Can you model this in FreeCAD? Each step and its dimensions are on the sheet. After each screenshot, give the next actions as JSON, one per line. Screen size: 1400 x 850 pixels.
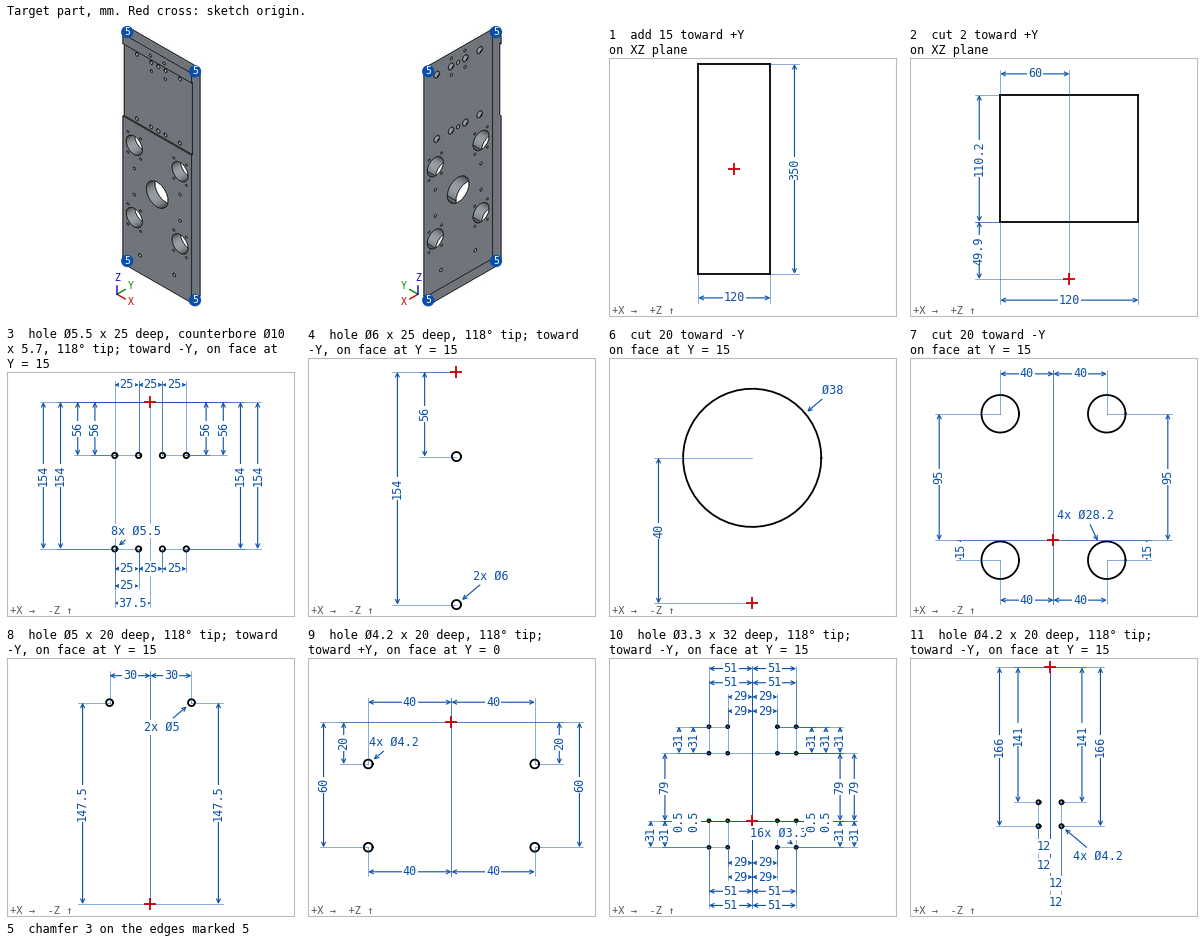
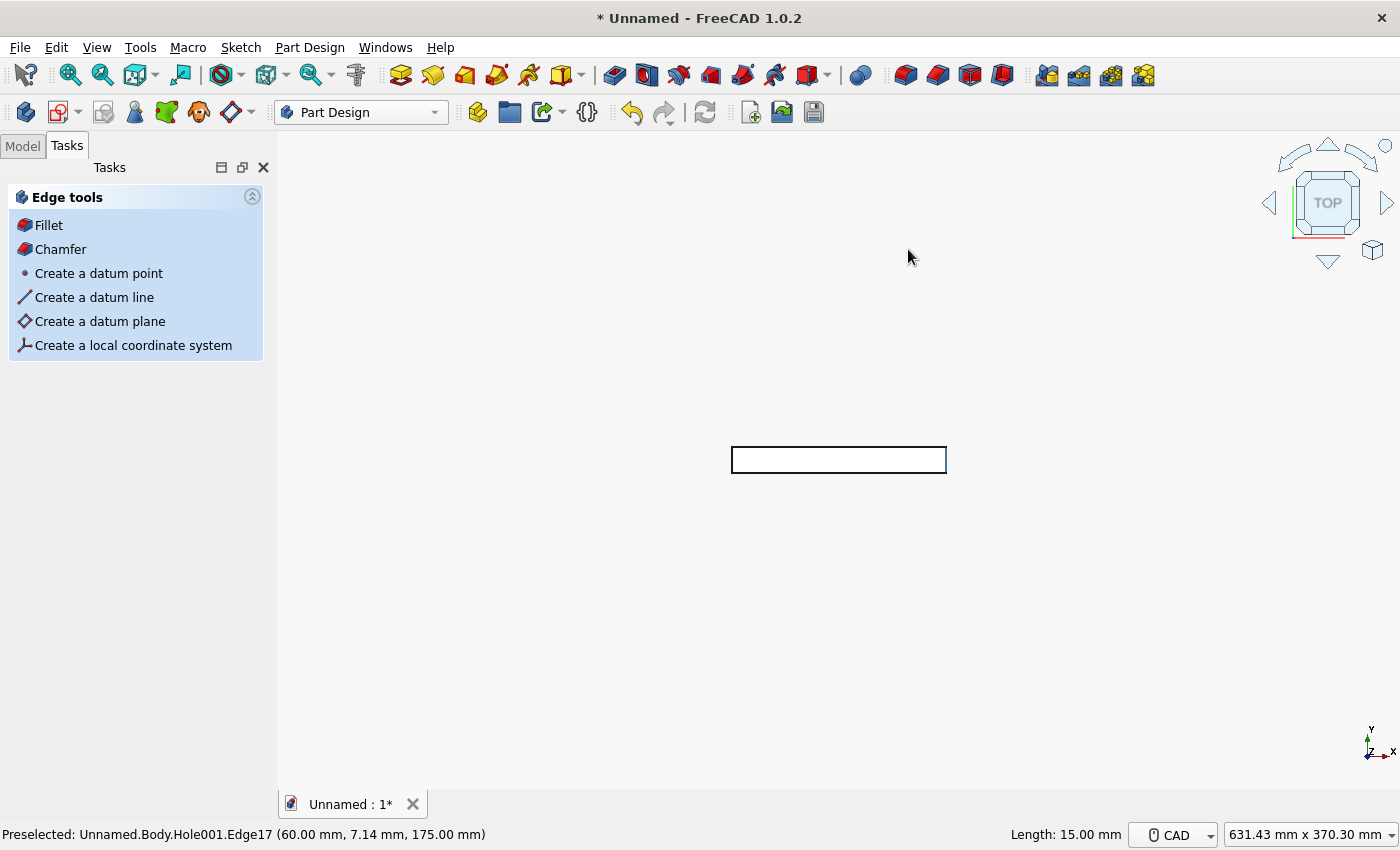
{"action": "key", "text": "v f"}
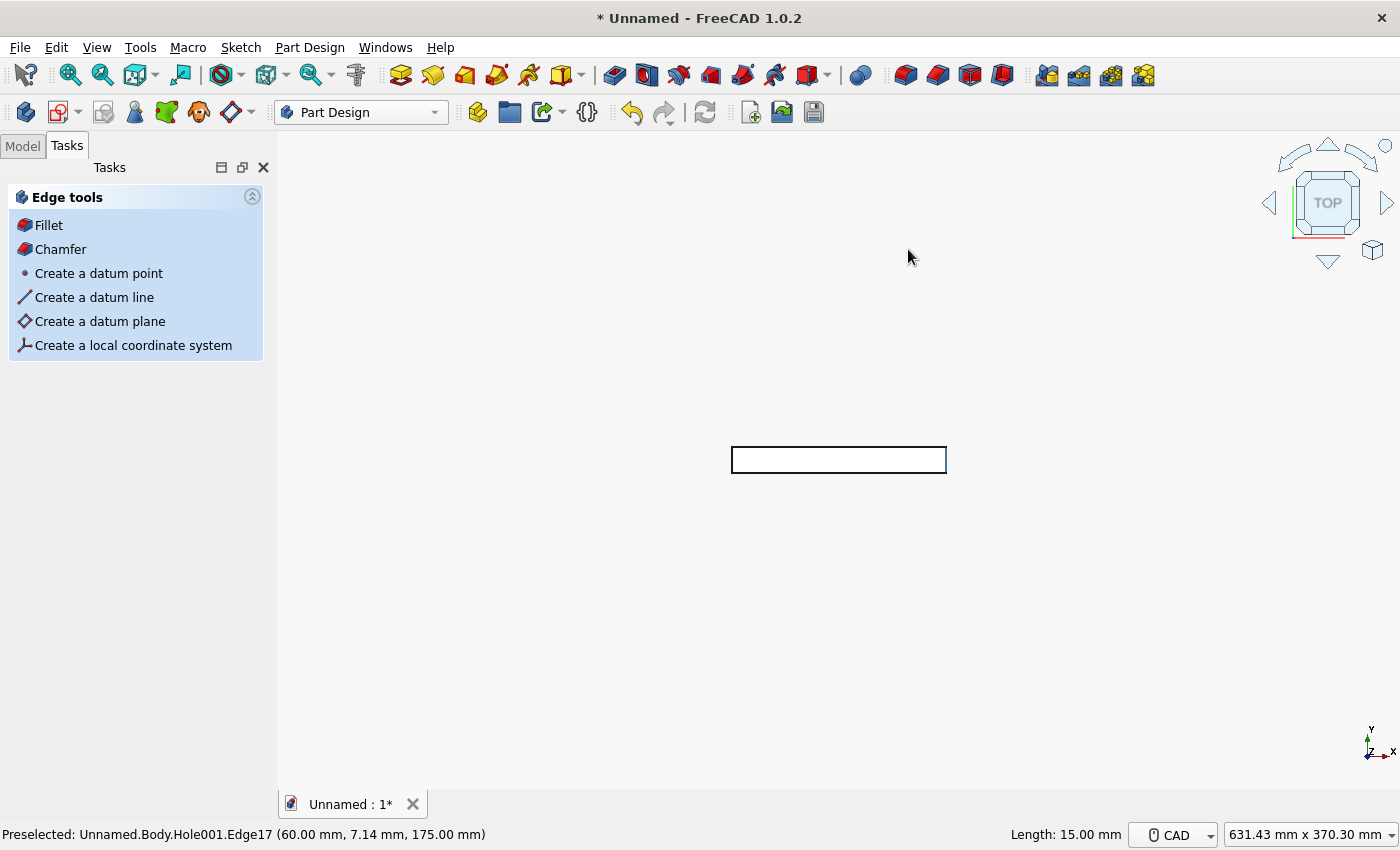
{"action": "left_click", "coordinate": [732, 459], "text": "ctrl"}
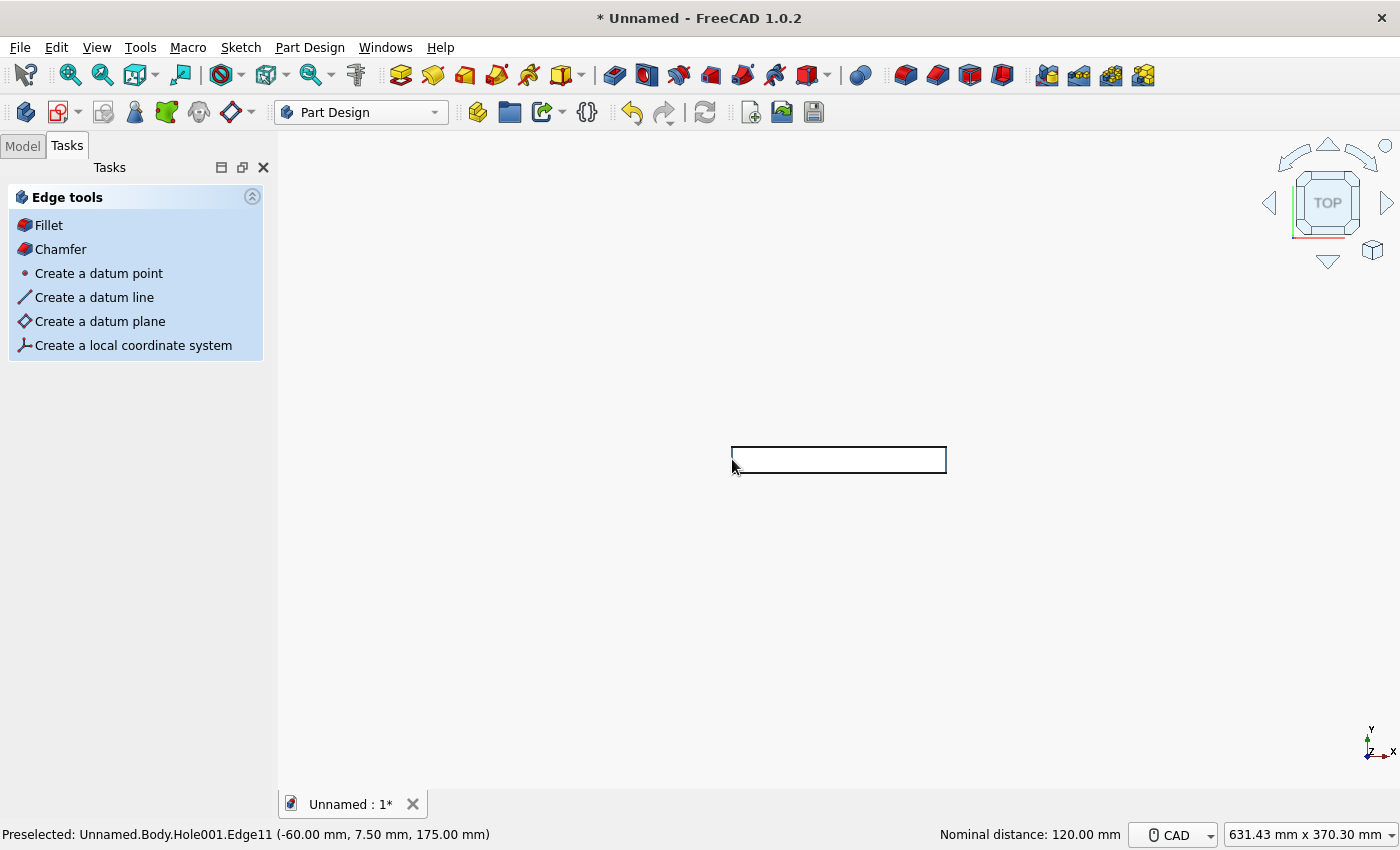
{"action": "key", "text": "1"}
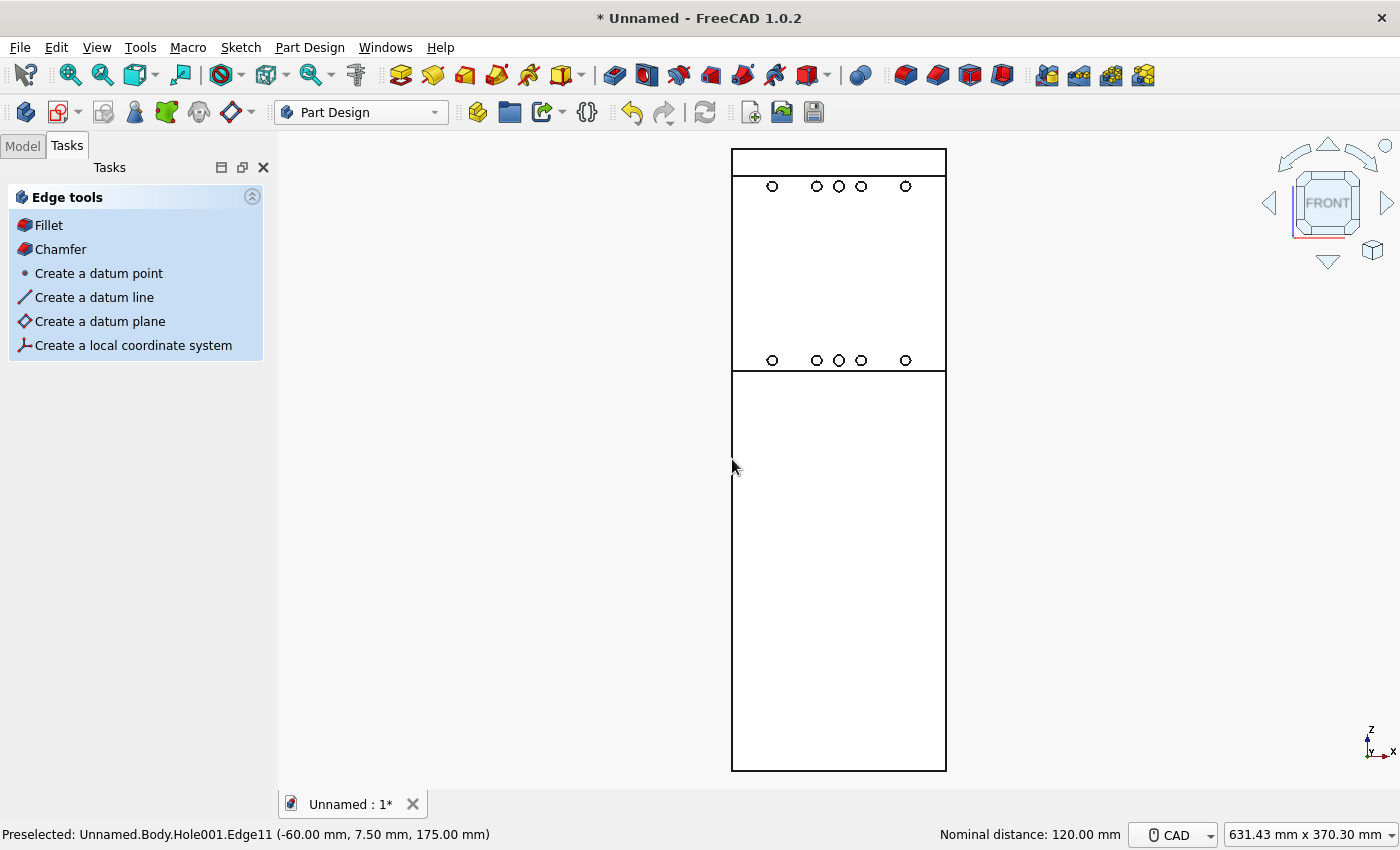
{"action": "key", "text": "3"}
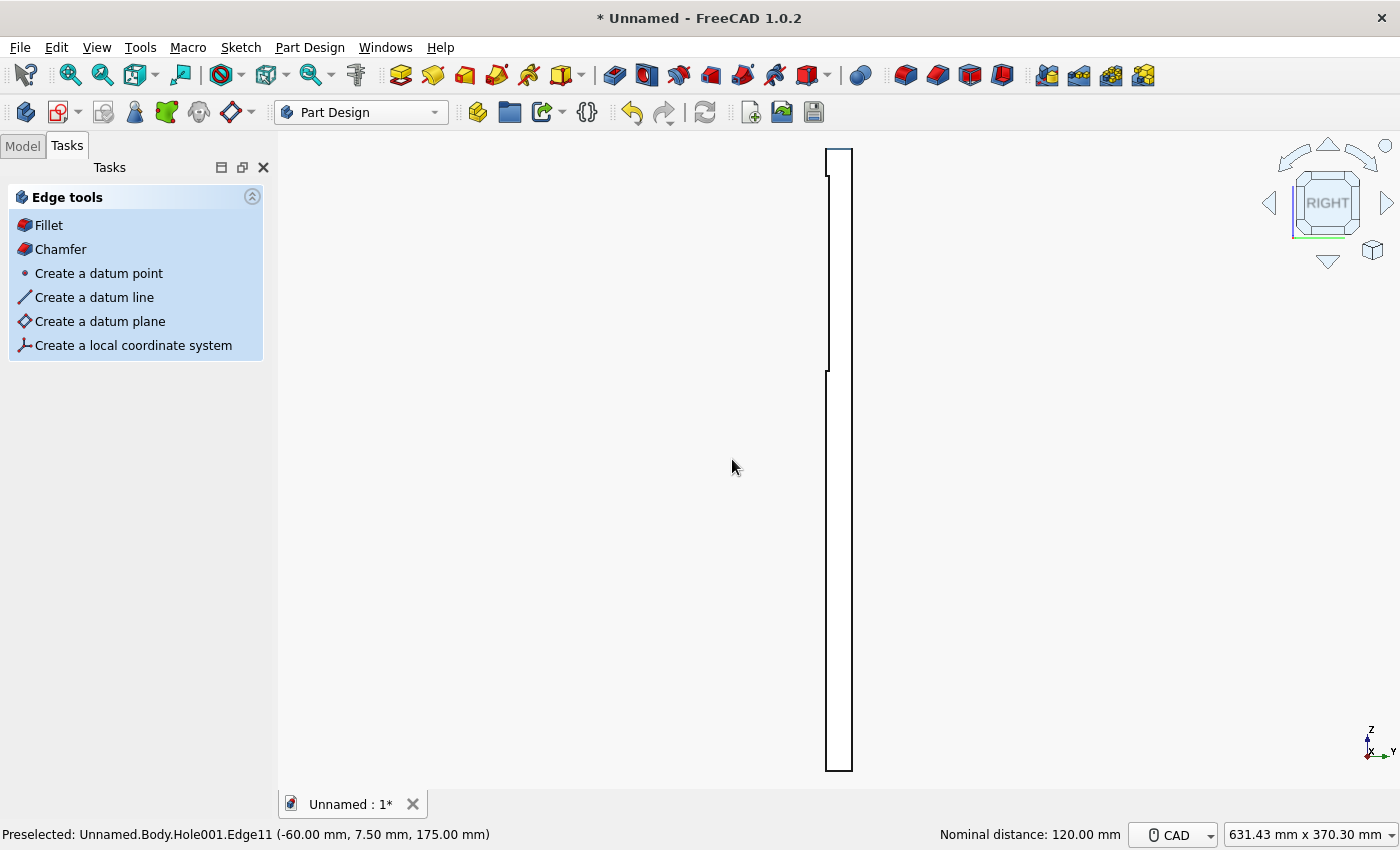
{"action": "key", "text": "5"}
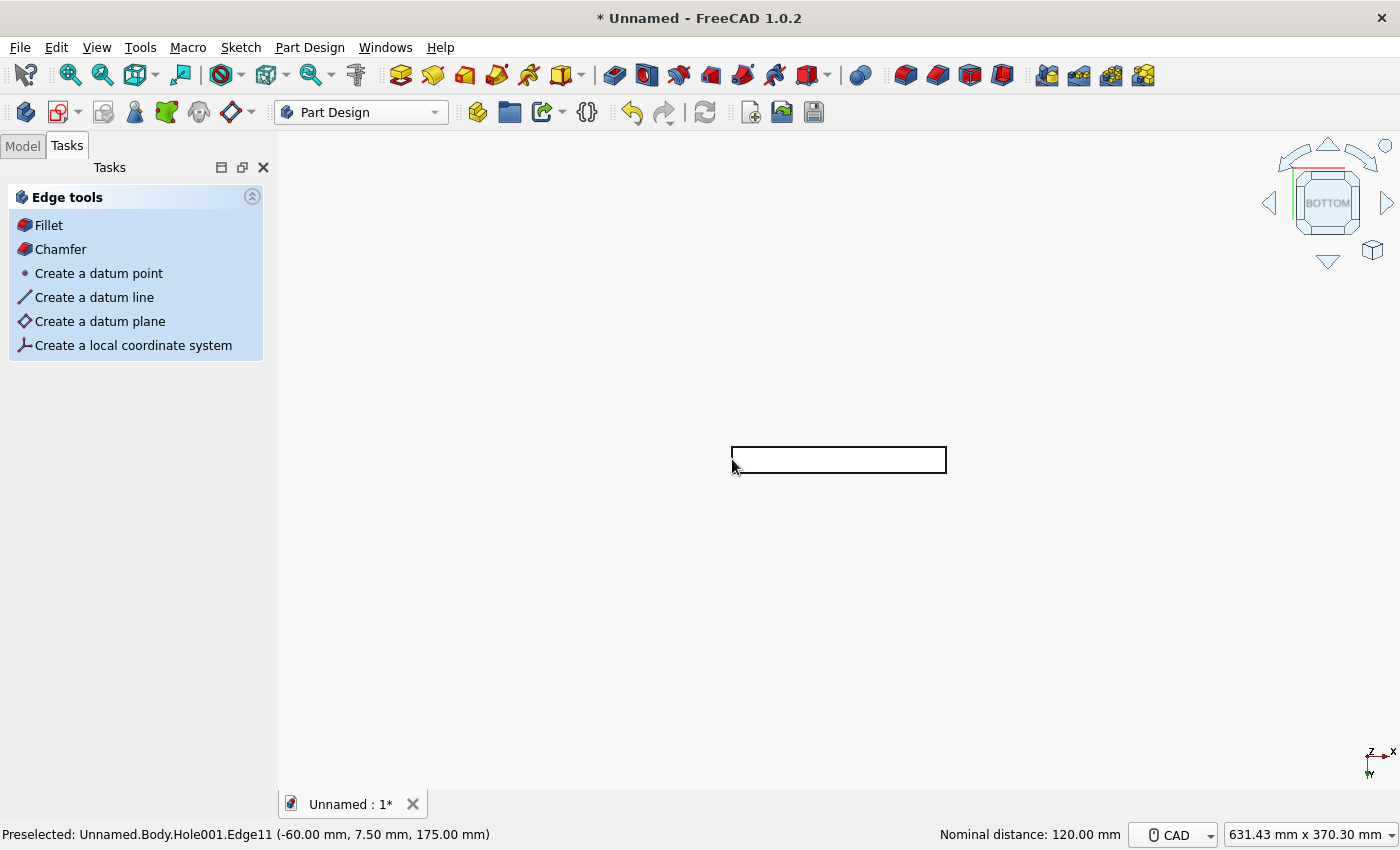
{"action": "left_click", "coordinate": [72, 76]}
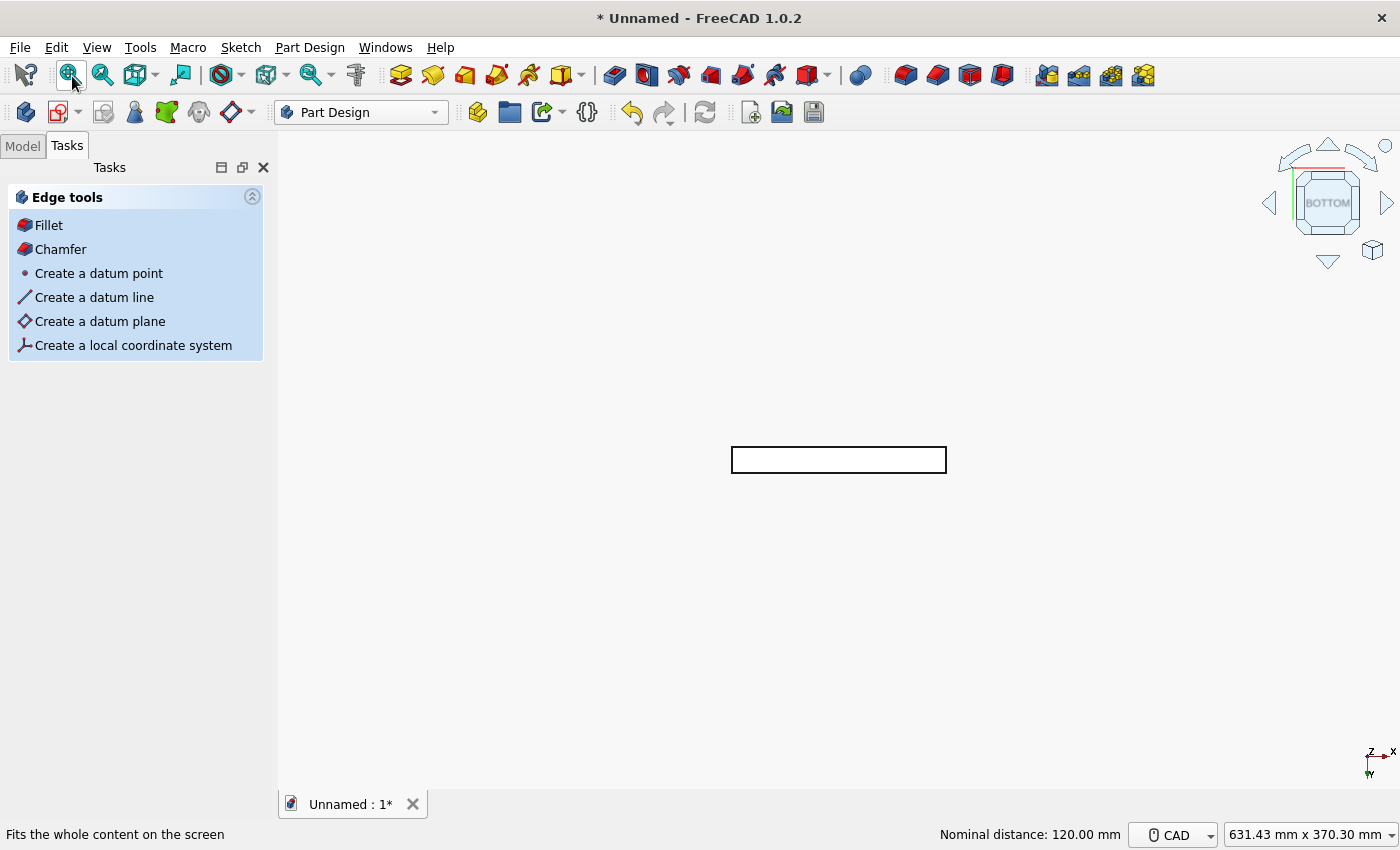
{"action": "left_click", "coordinate": [732, 459], "text": "ctrl"}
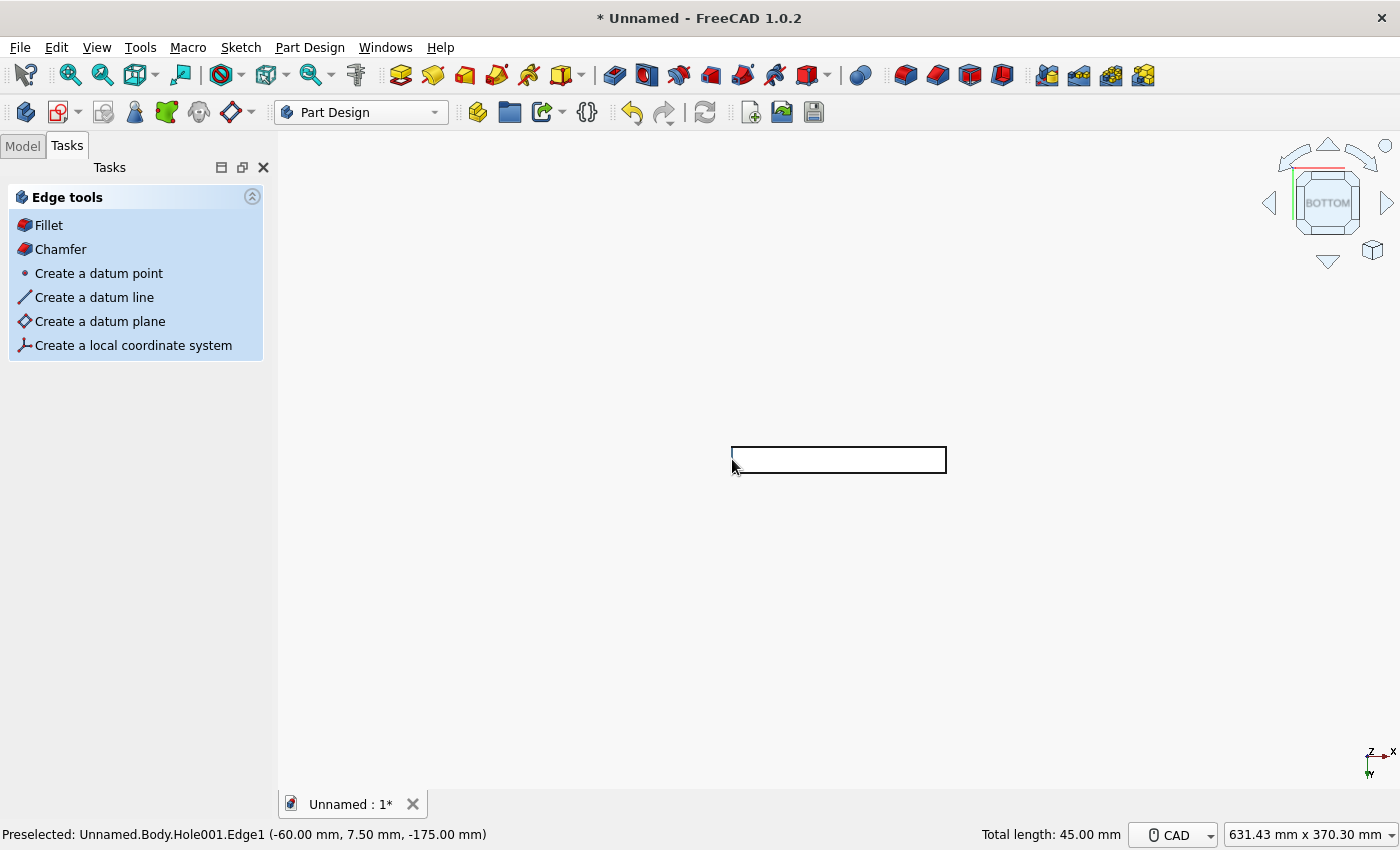
{"action": "left_click", "coordinate": [946, 459], "text": "ctrl"}